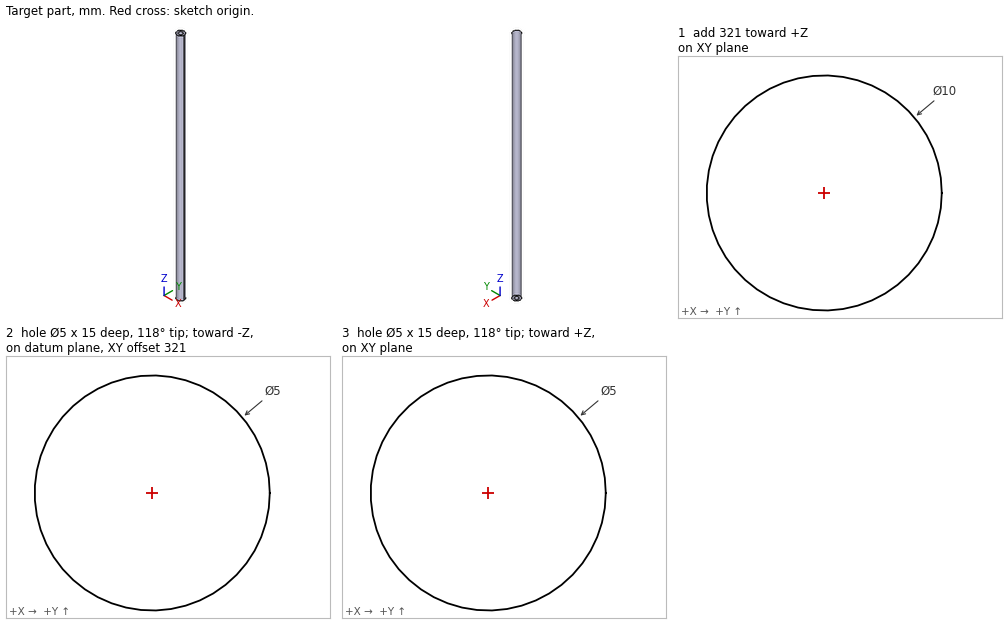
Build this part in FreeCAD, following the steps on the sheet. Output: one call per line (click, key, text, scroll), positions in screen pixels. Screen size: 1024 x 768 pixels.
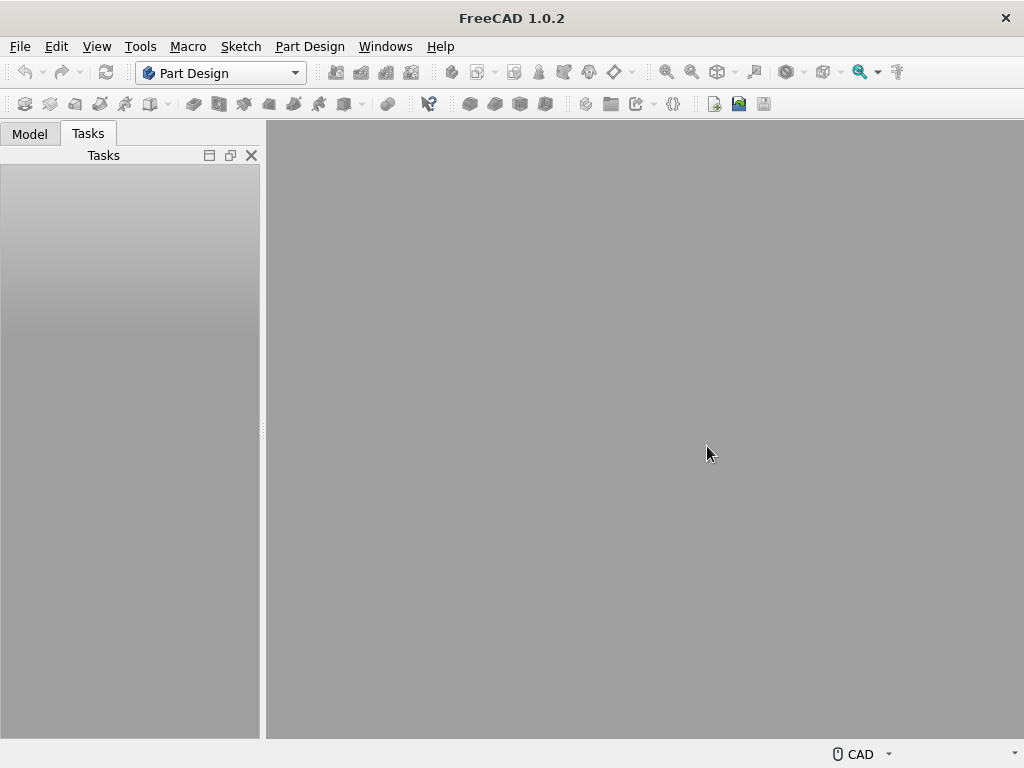
click(714, 104)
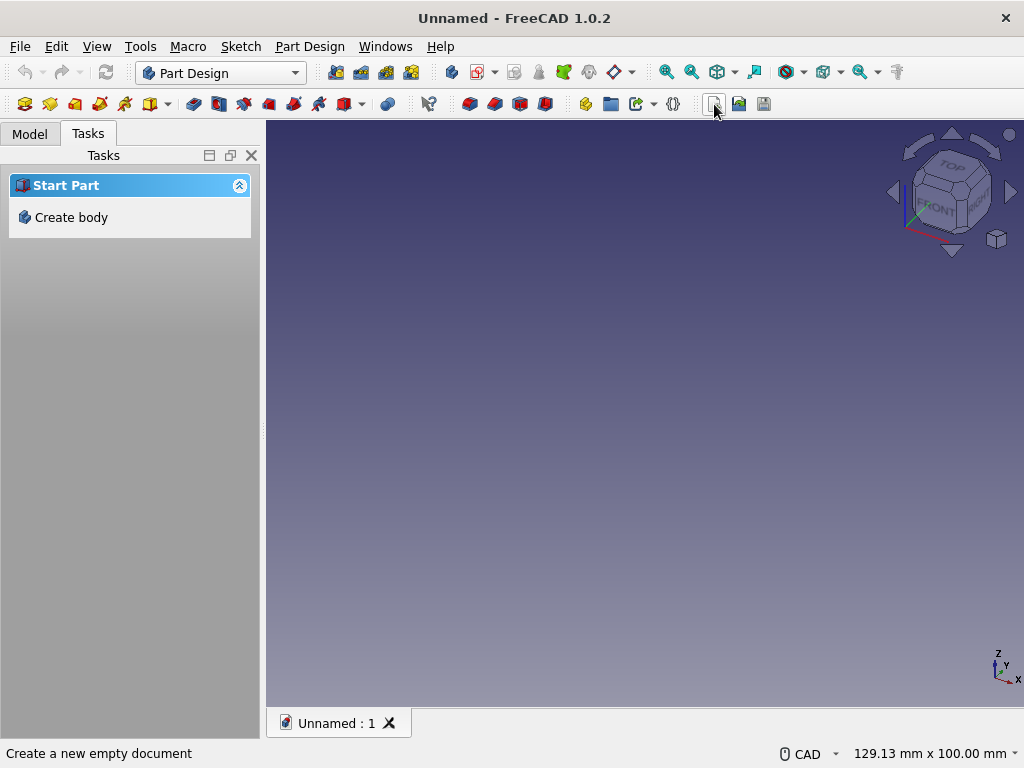
click(476, 72)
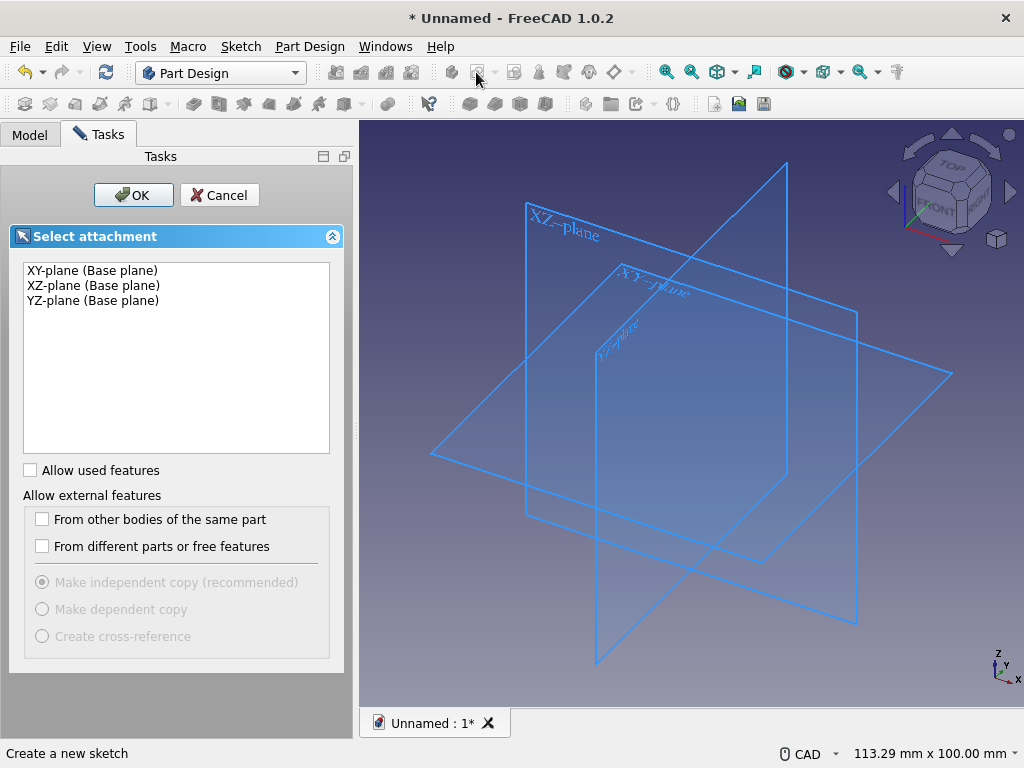
click(84, 270)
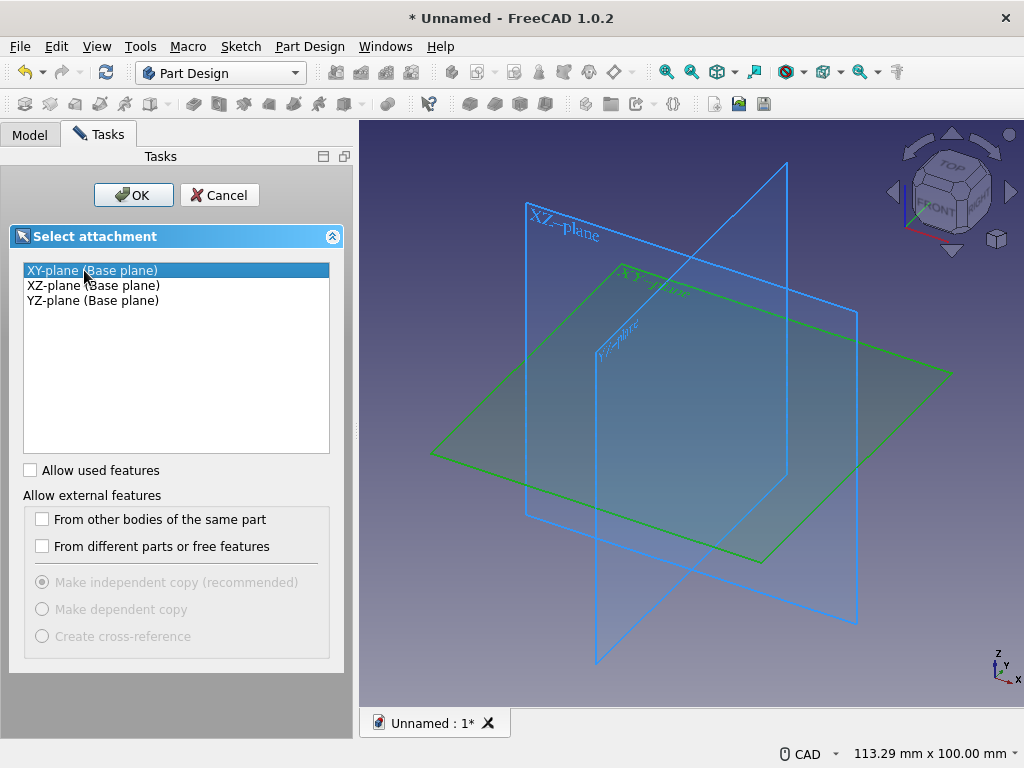
click(134, 195)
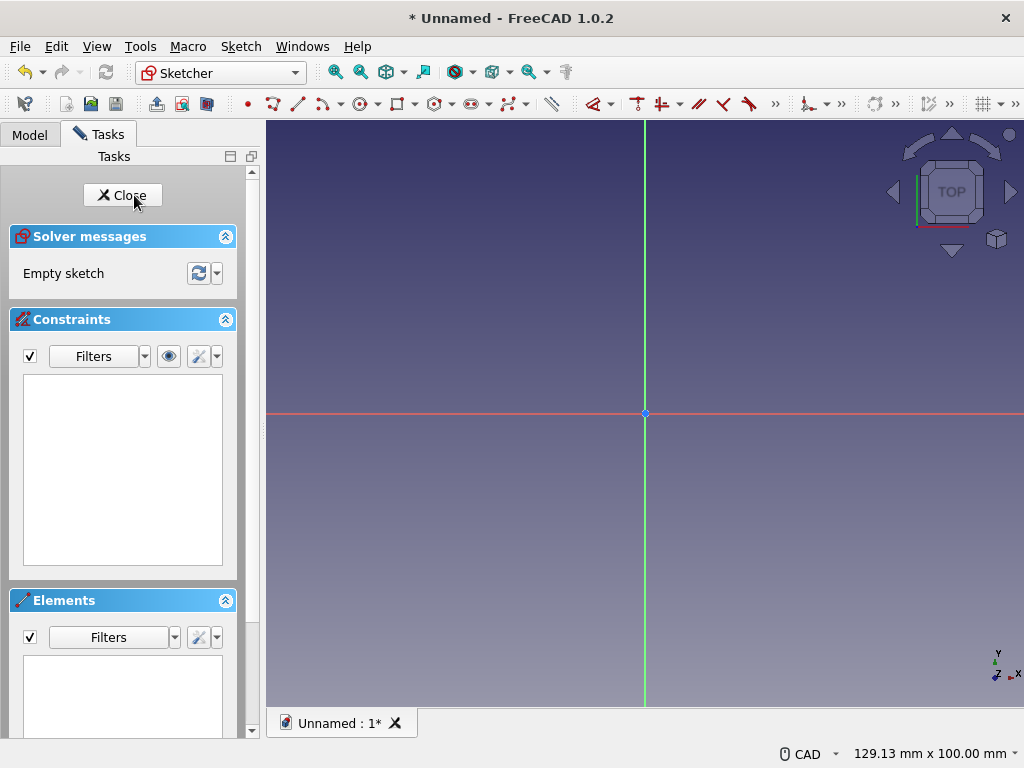
scroll(659, 414, up, 9)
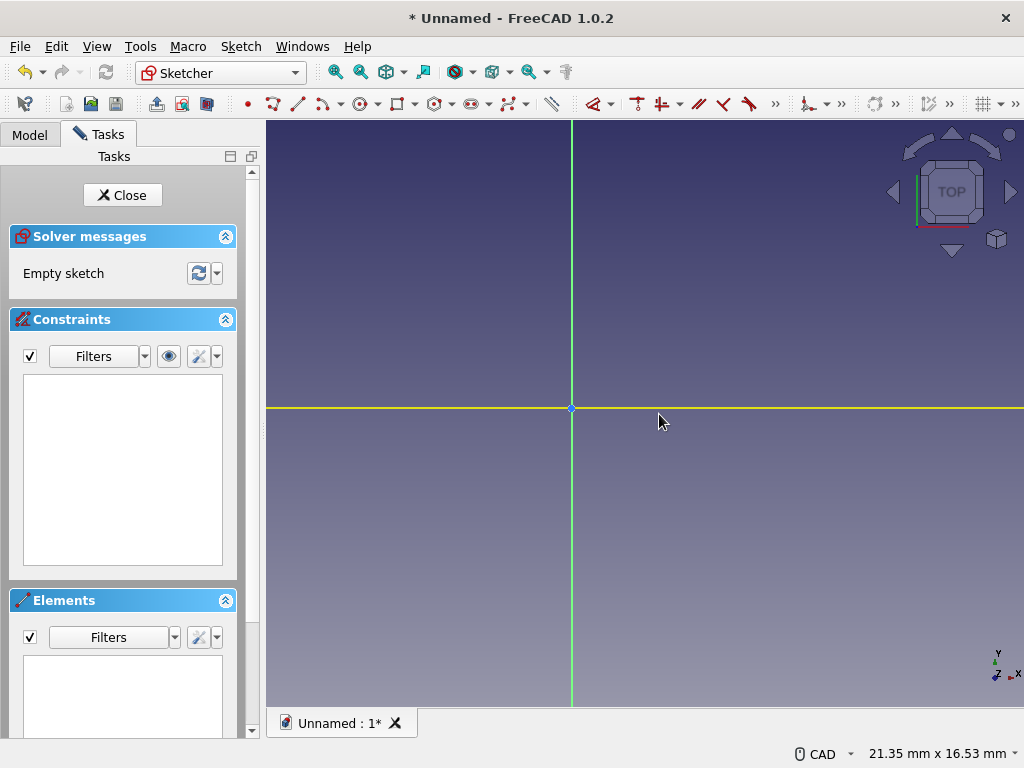
click(360, 104)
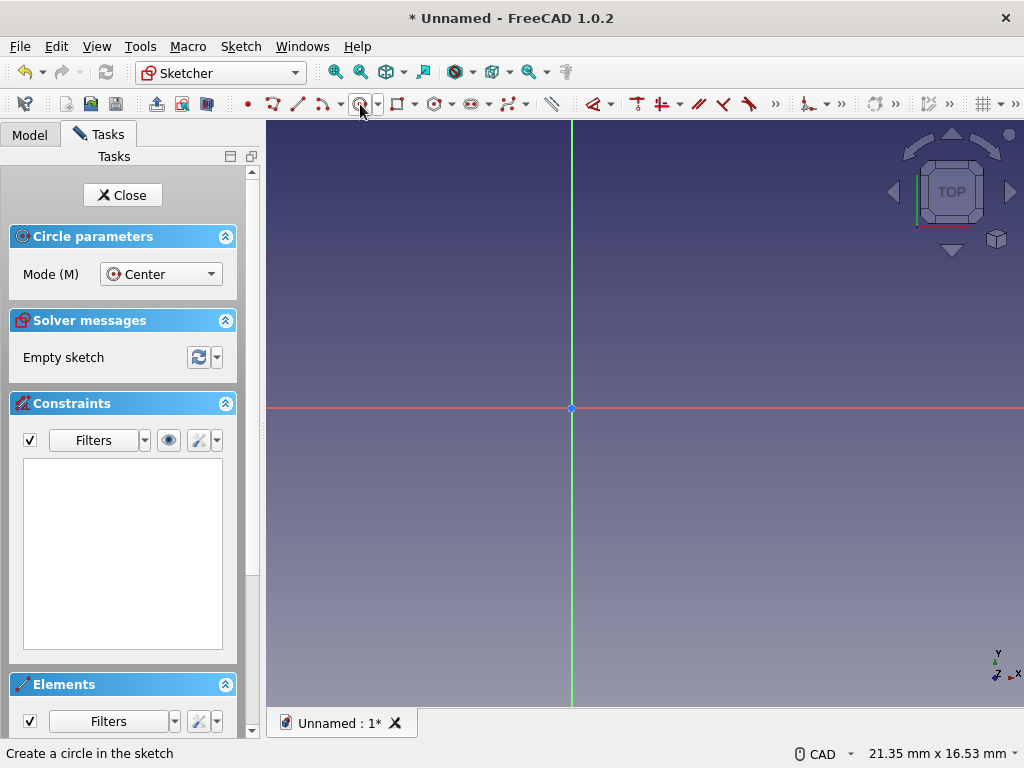
click(572, 408)
move(697, 283)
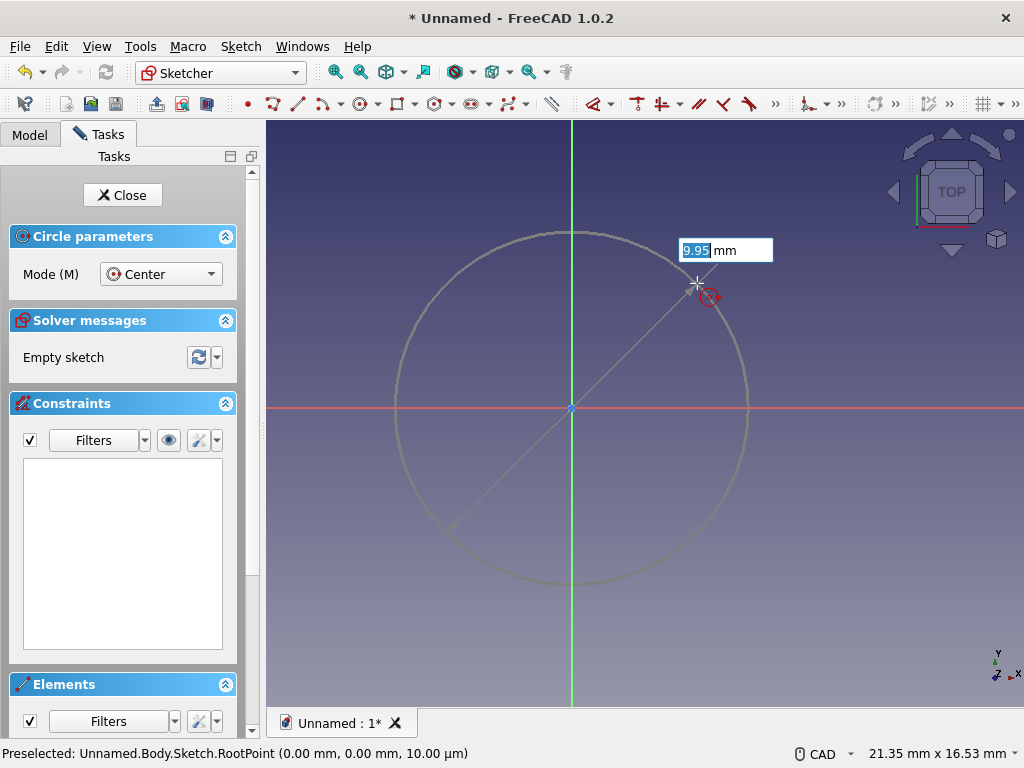
text(10)
key(Return)
key(Escape)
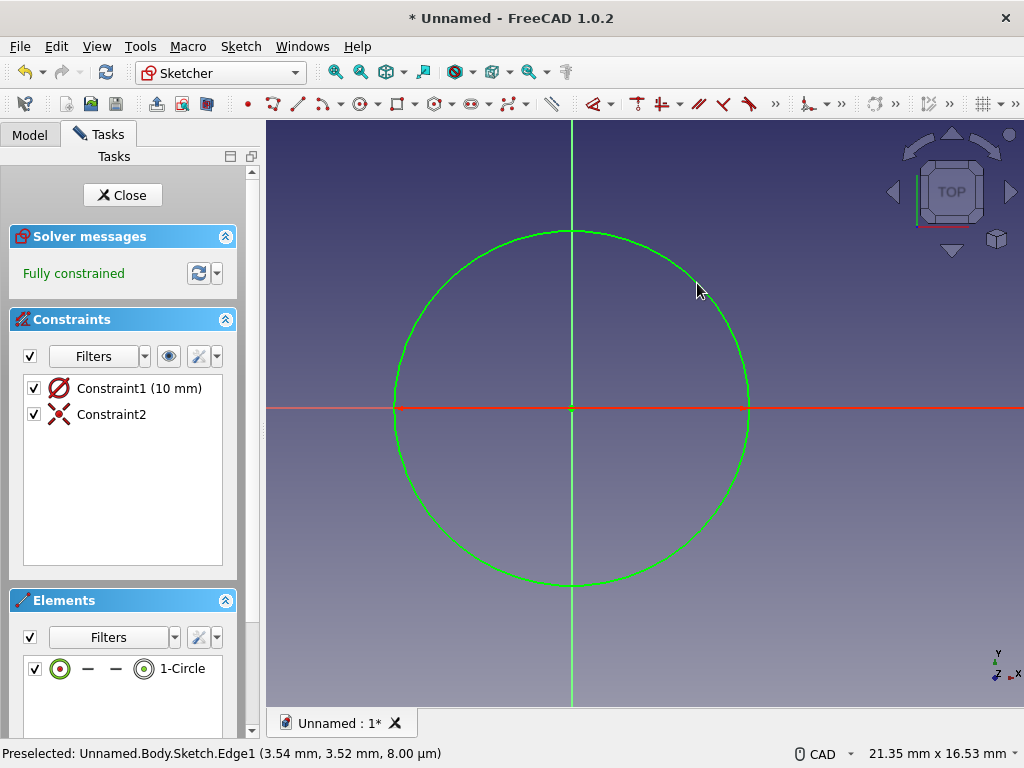
click(123, 195)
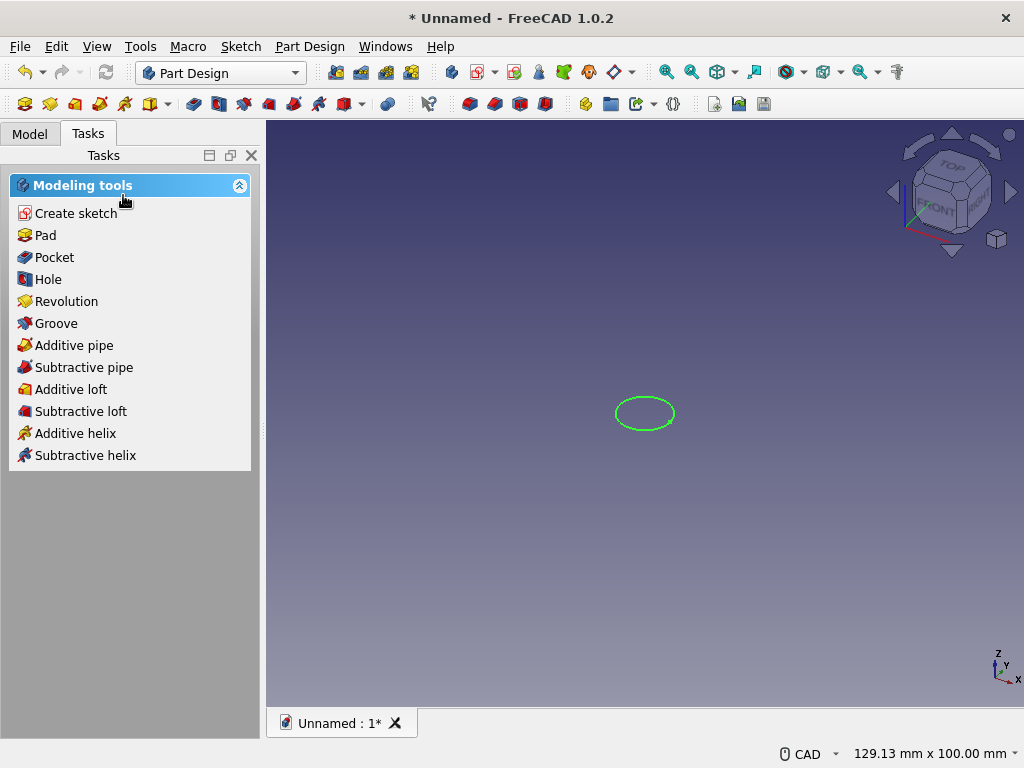
click(25, 104)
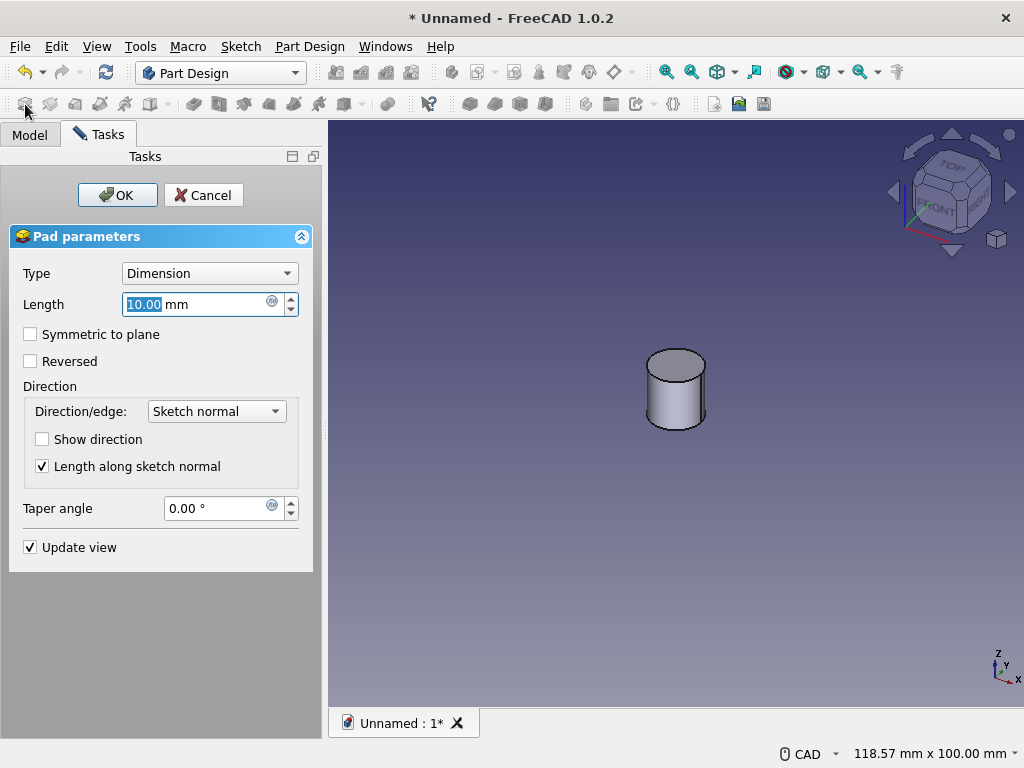
text(321)
key(Tab)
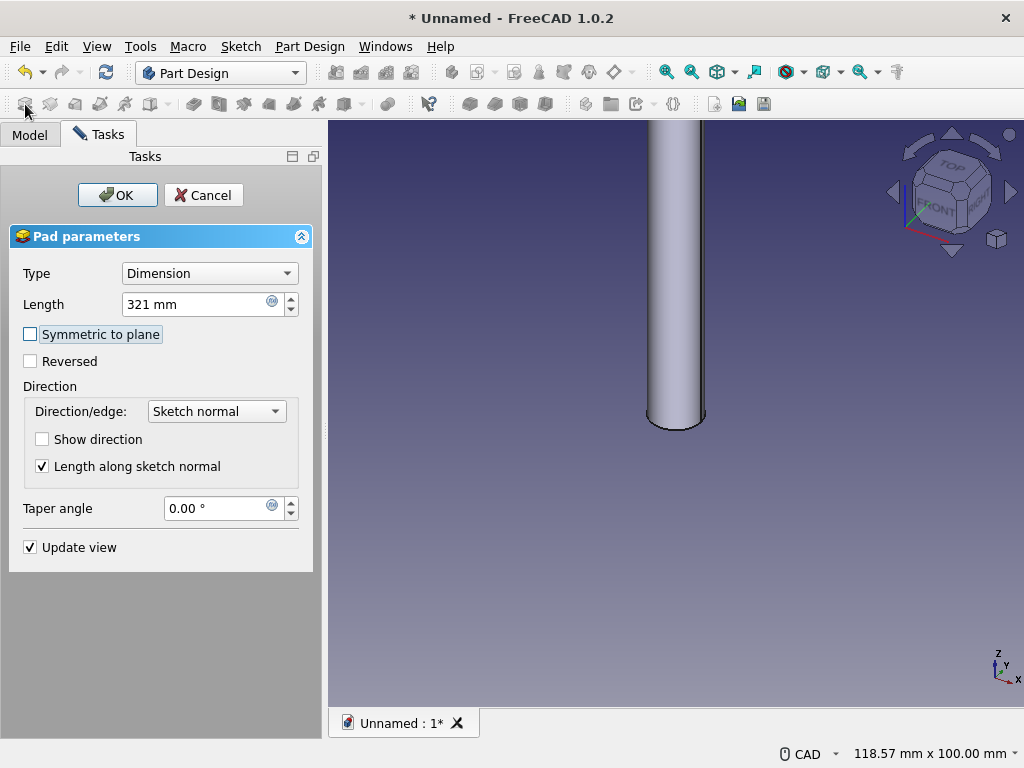
click(118, 195)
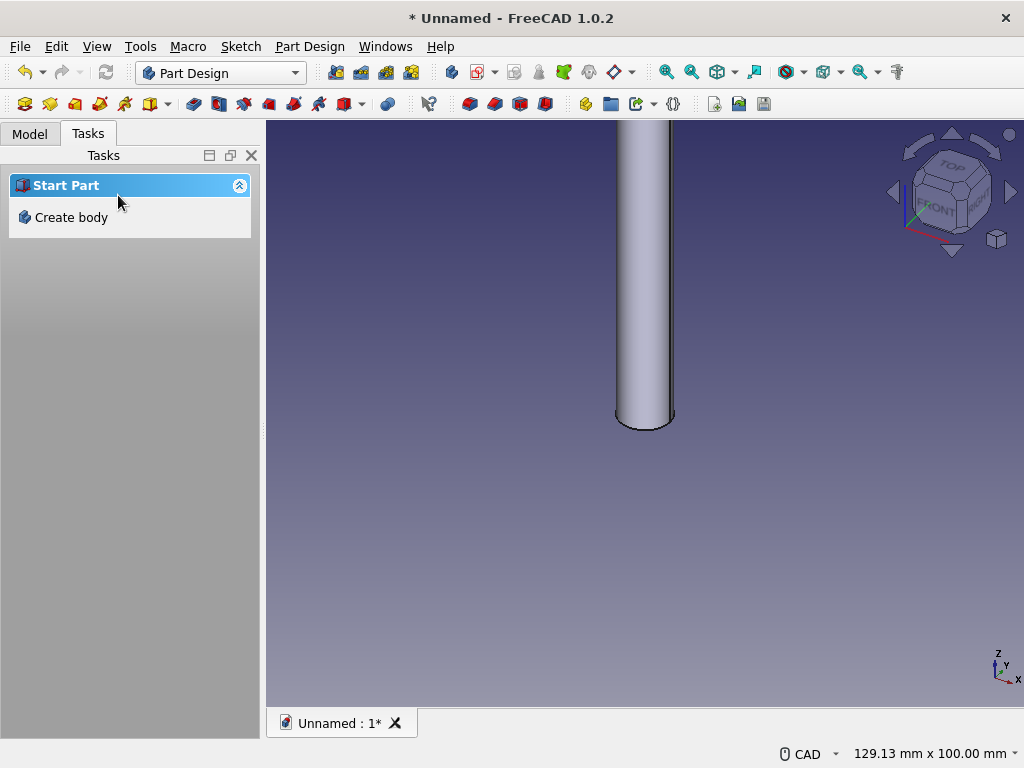
click(667, 72)